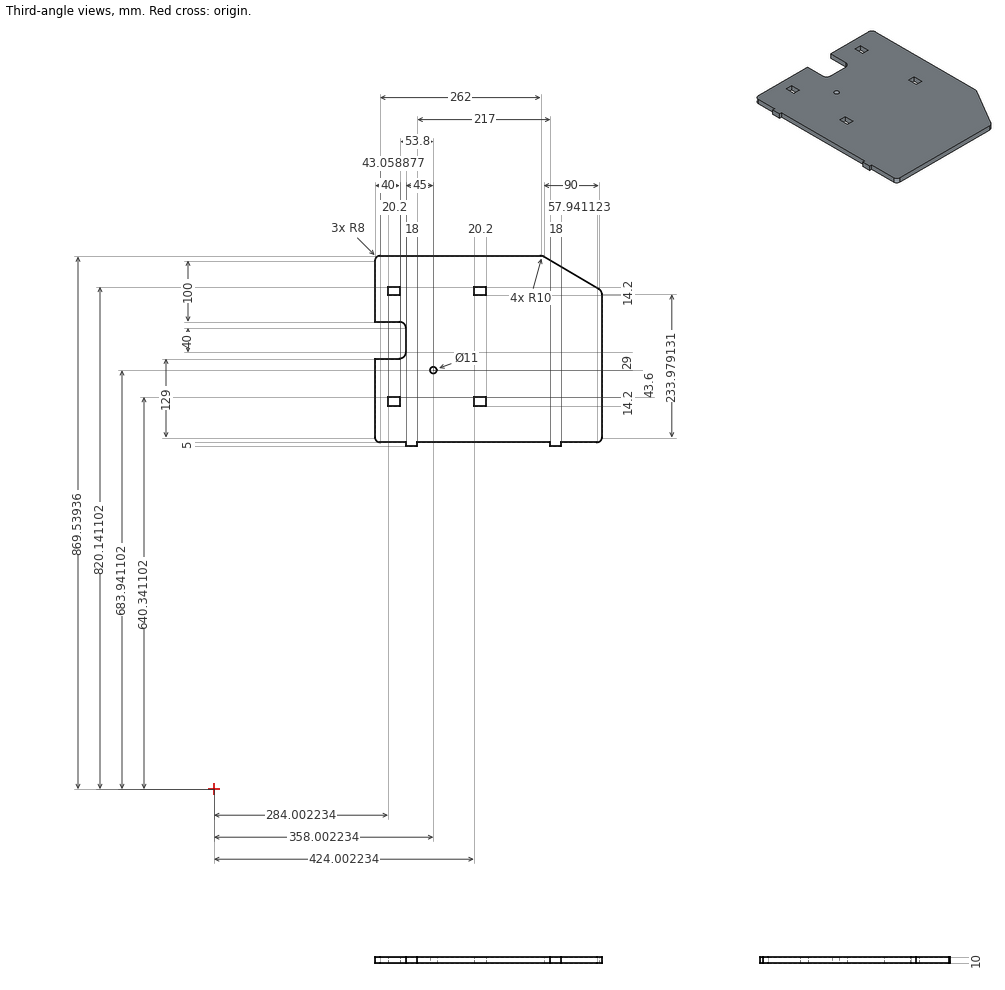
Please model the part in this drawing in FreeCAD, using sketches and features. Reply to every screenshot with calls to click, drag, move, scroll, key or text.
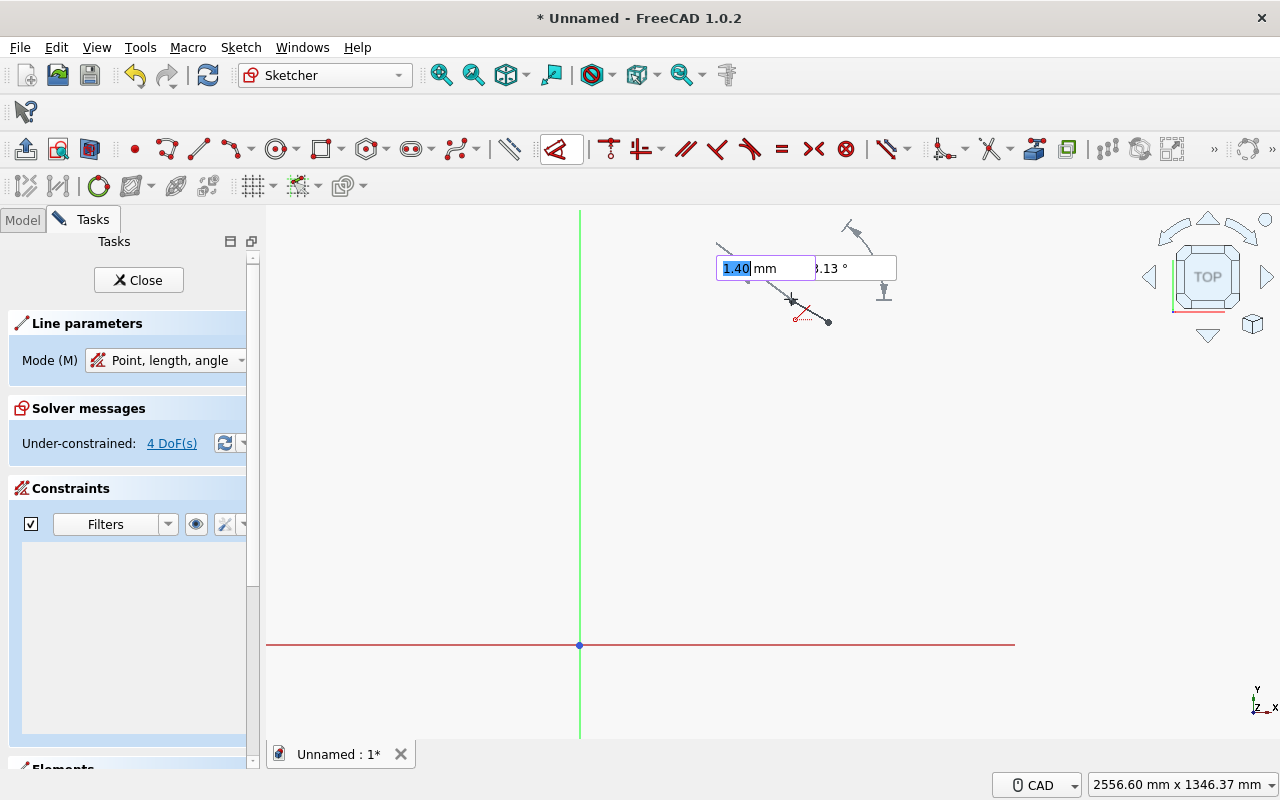
click(687, 300)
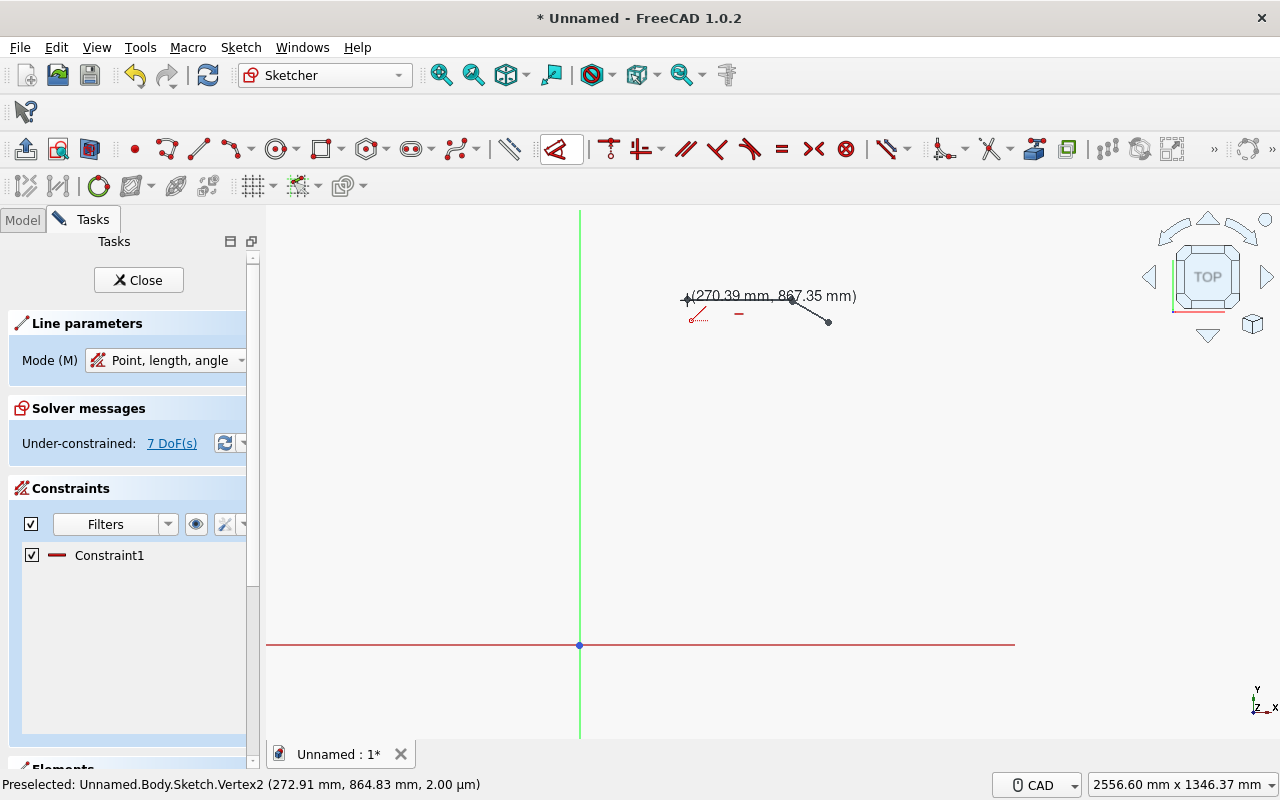
click(168, 150)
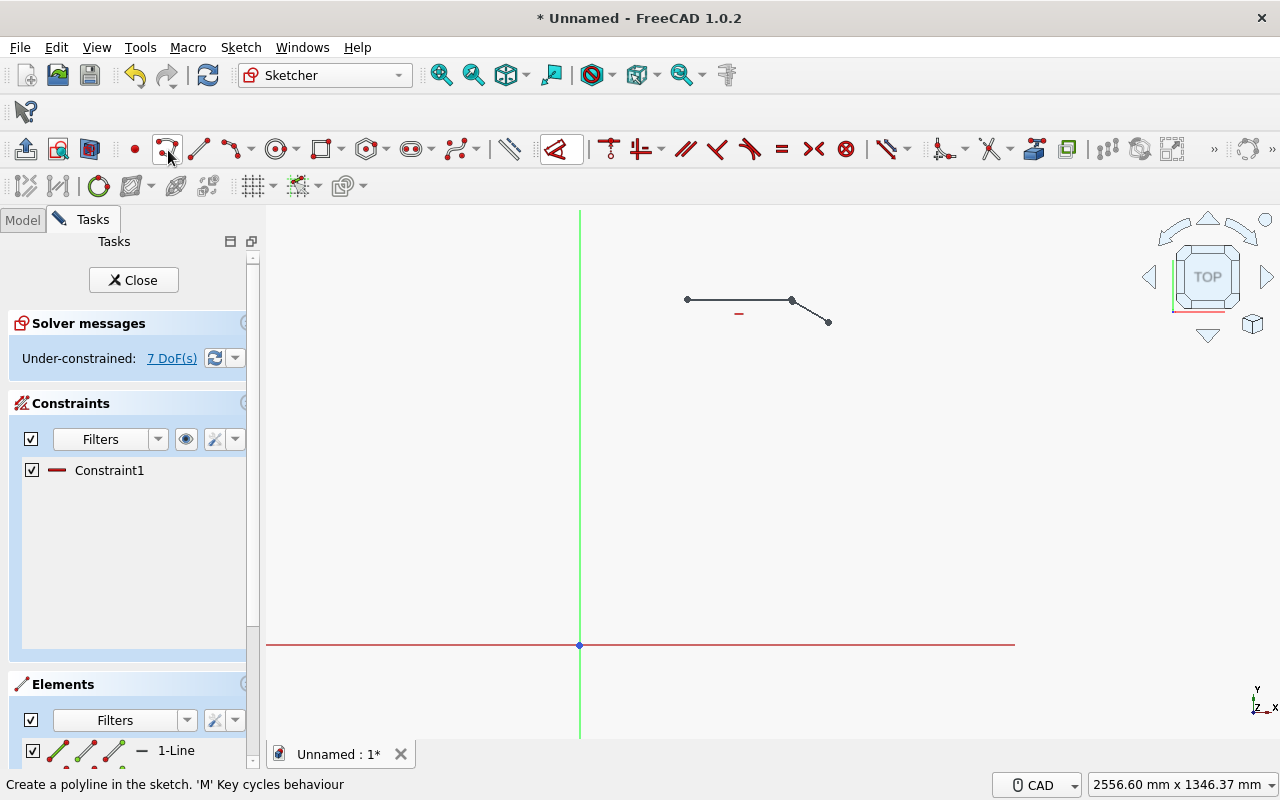
scroll(684, 303, up, 7)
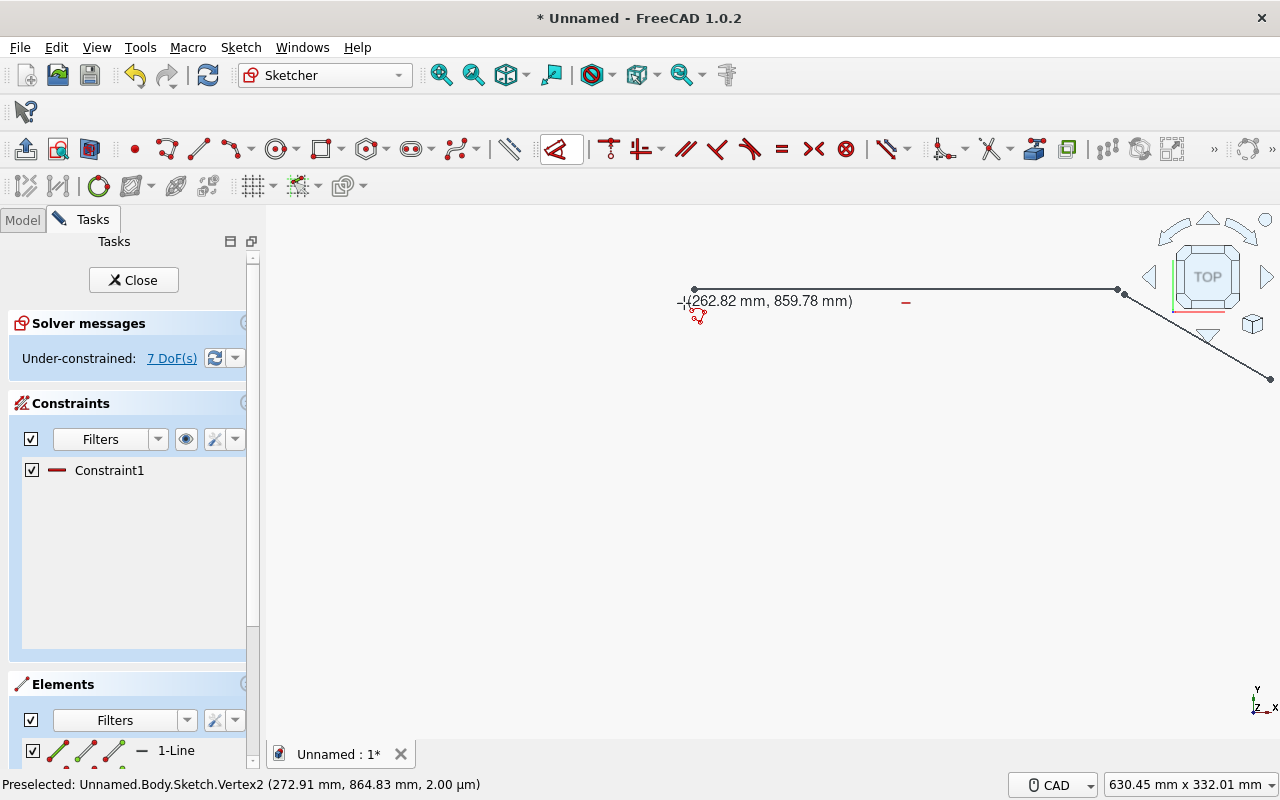
click(683, 301)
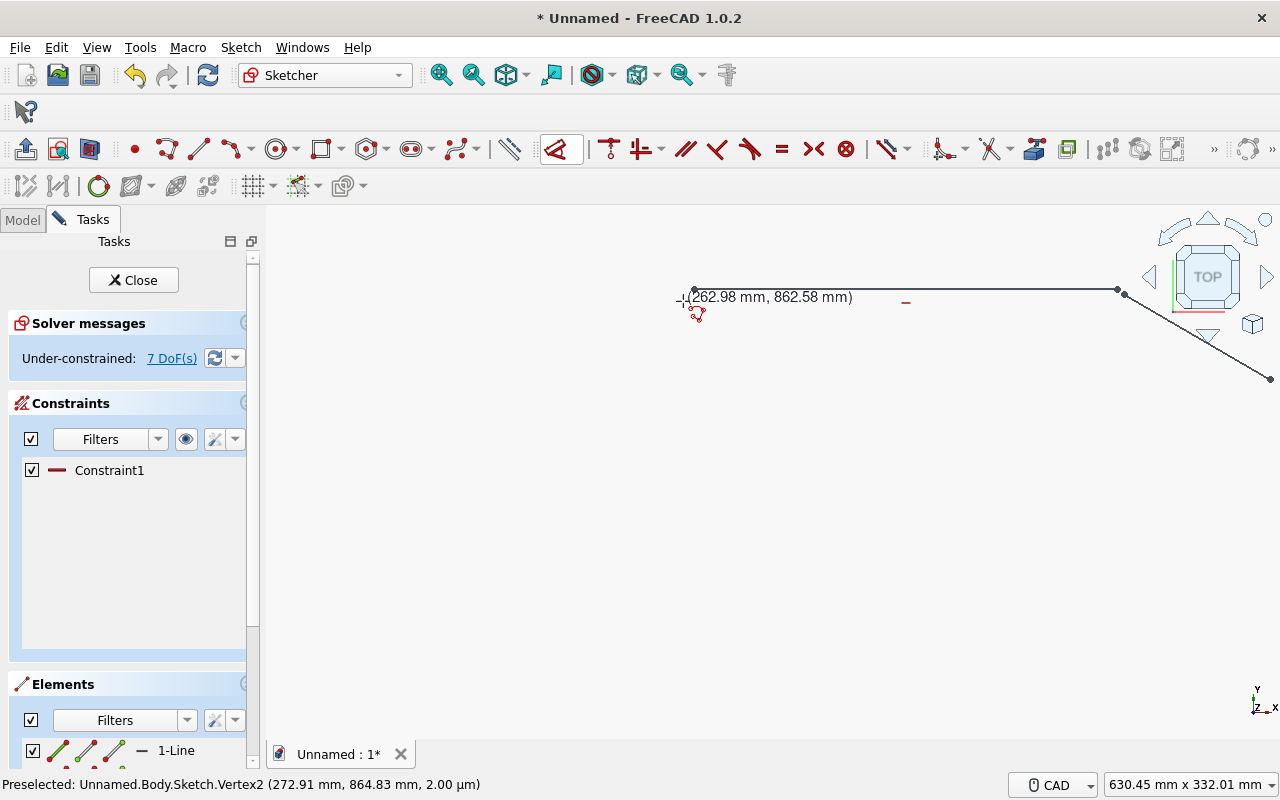
scroll(683, 303, down, 7)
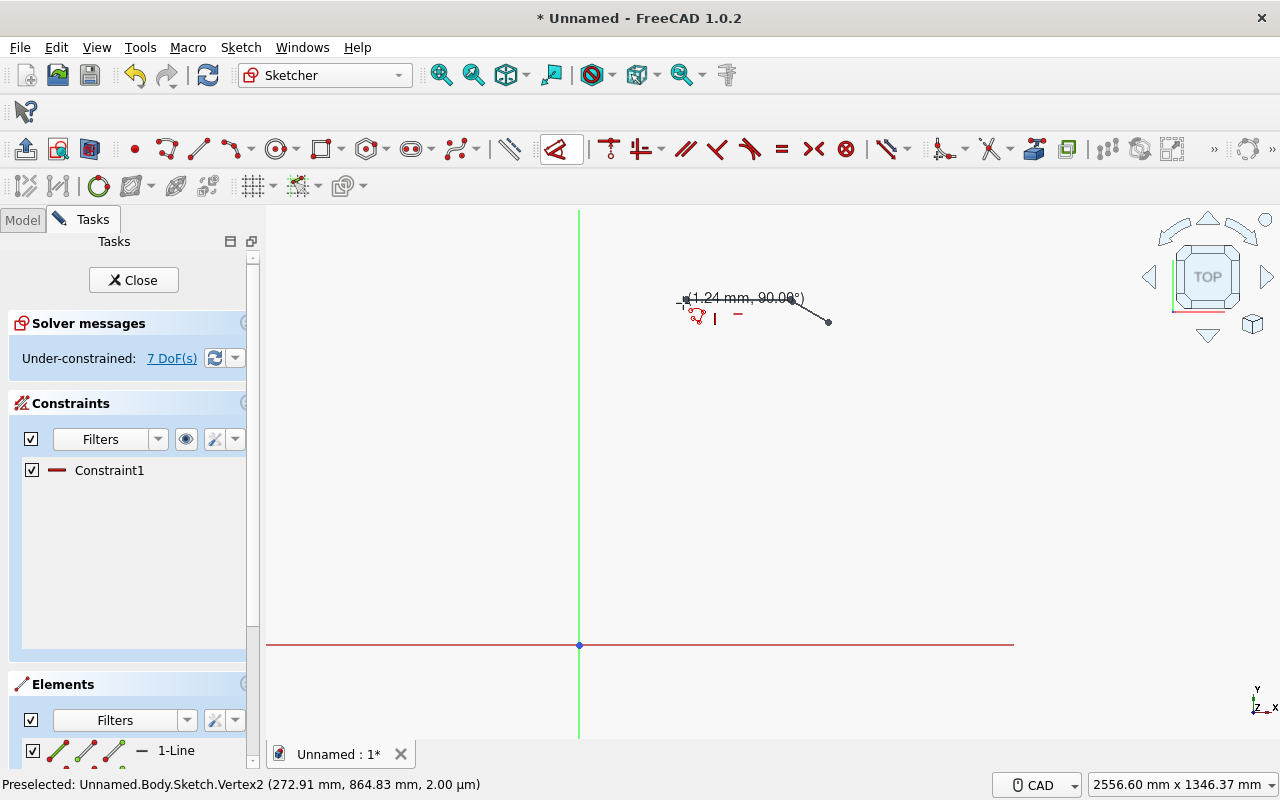
click(683, 342)
click(699, 342)
right_click(699, 342)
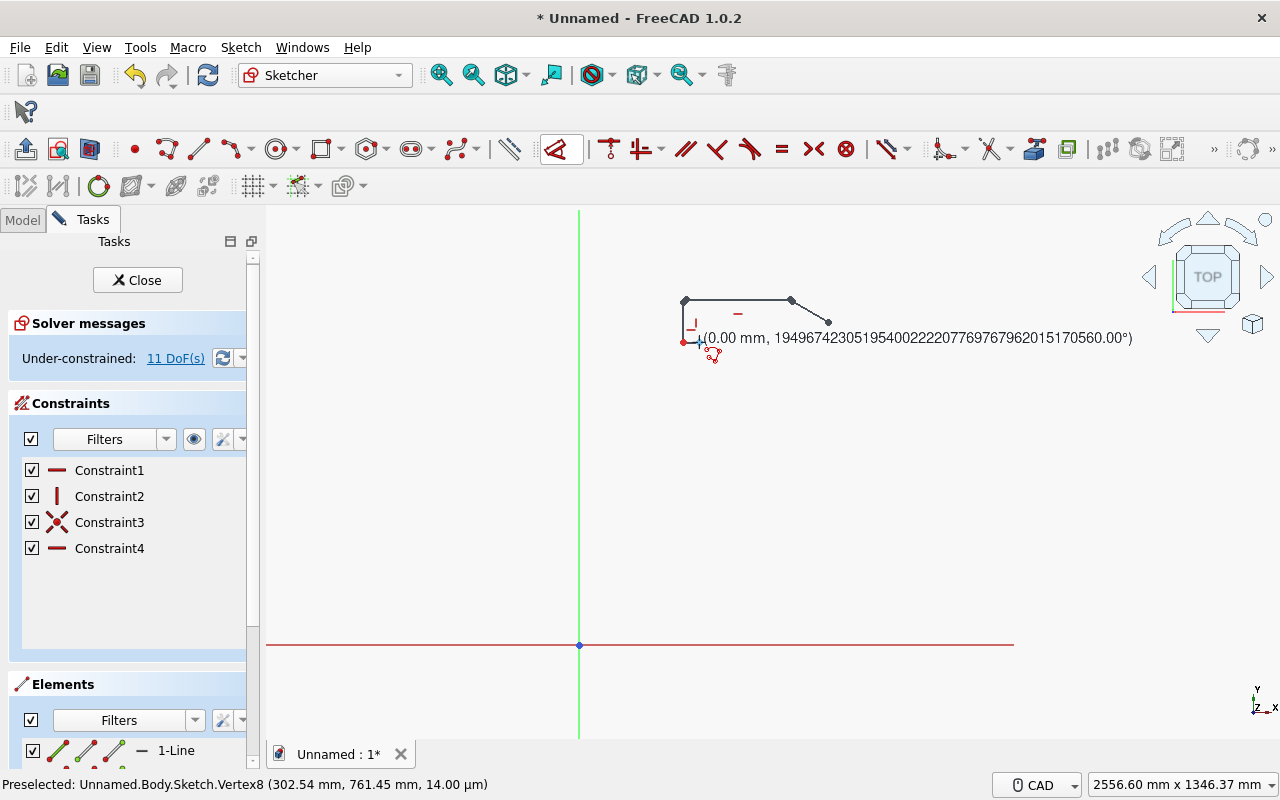
key(g)
key(l)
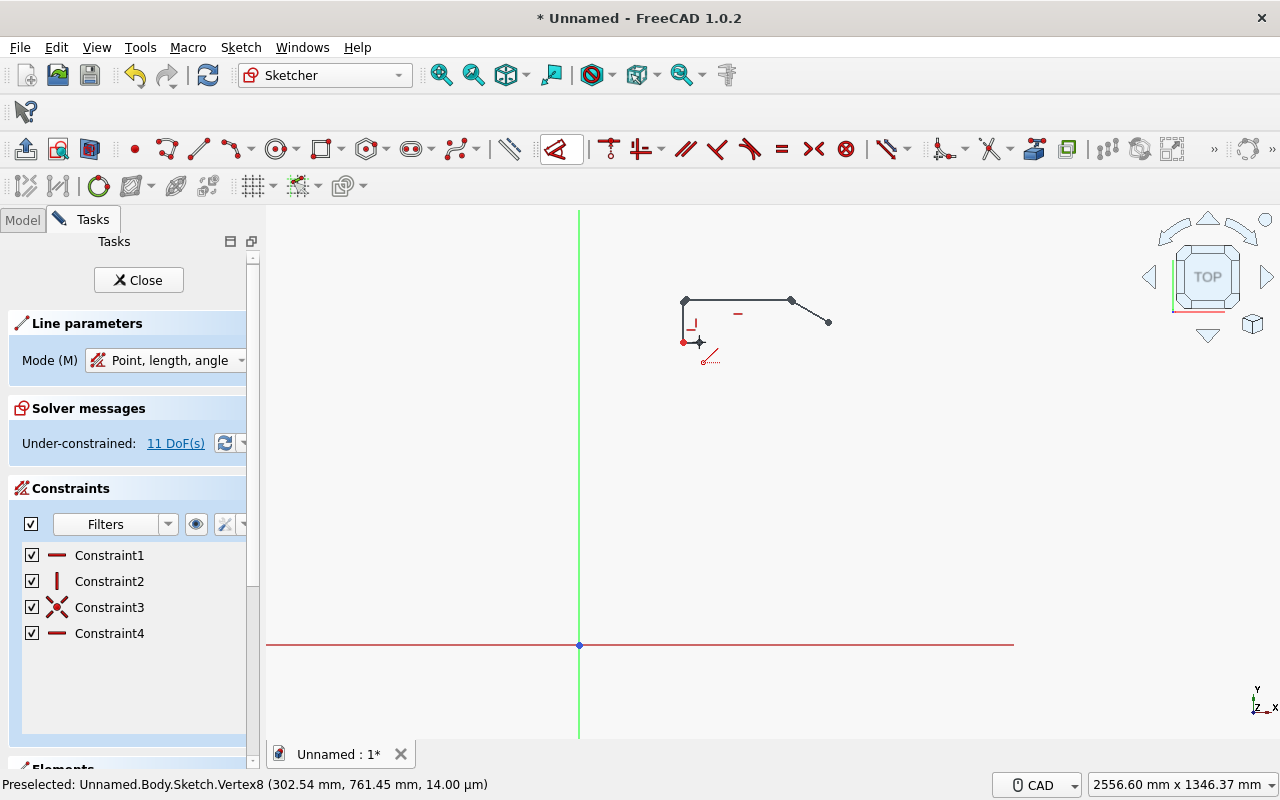
scroll(703, 346, up, 6)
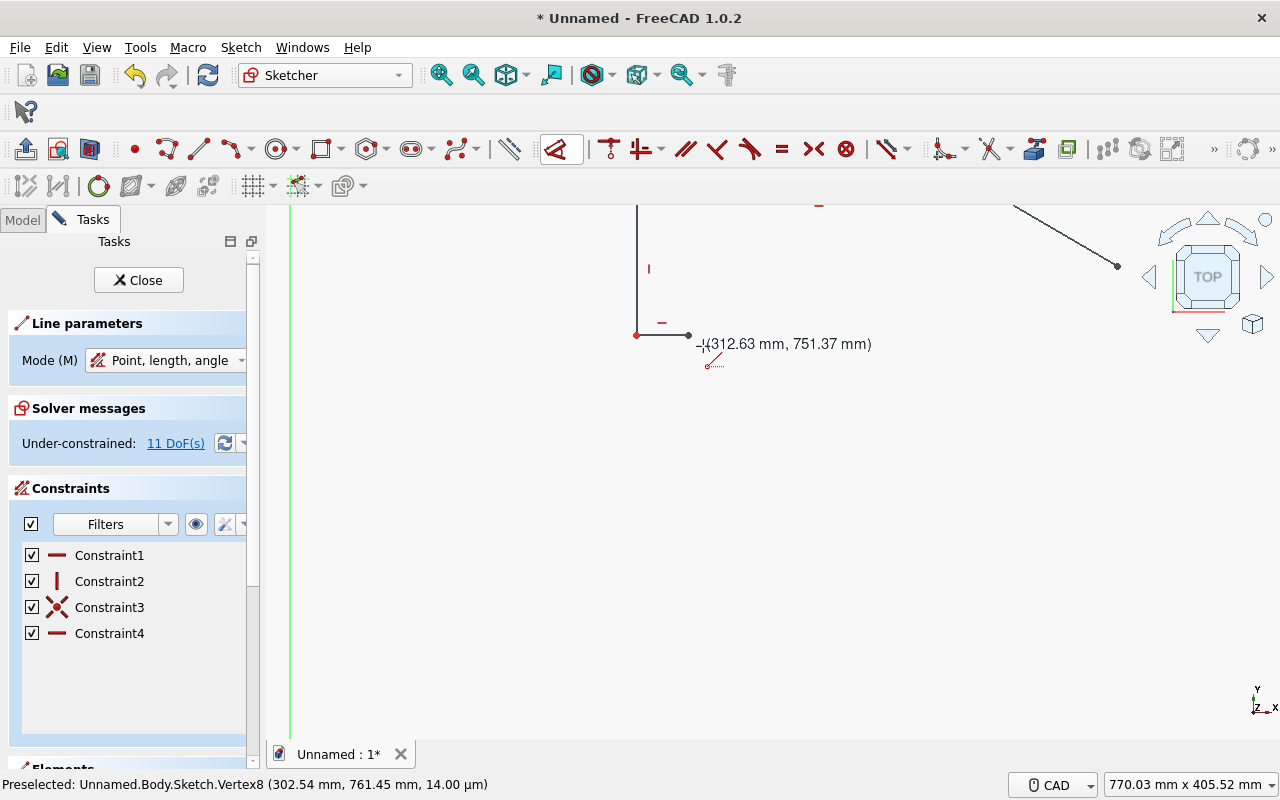
click(702, 347)
click(702, 399)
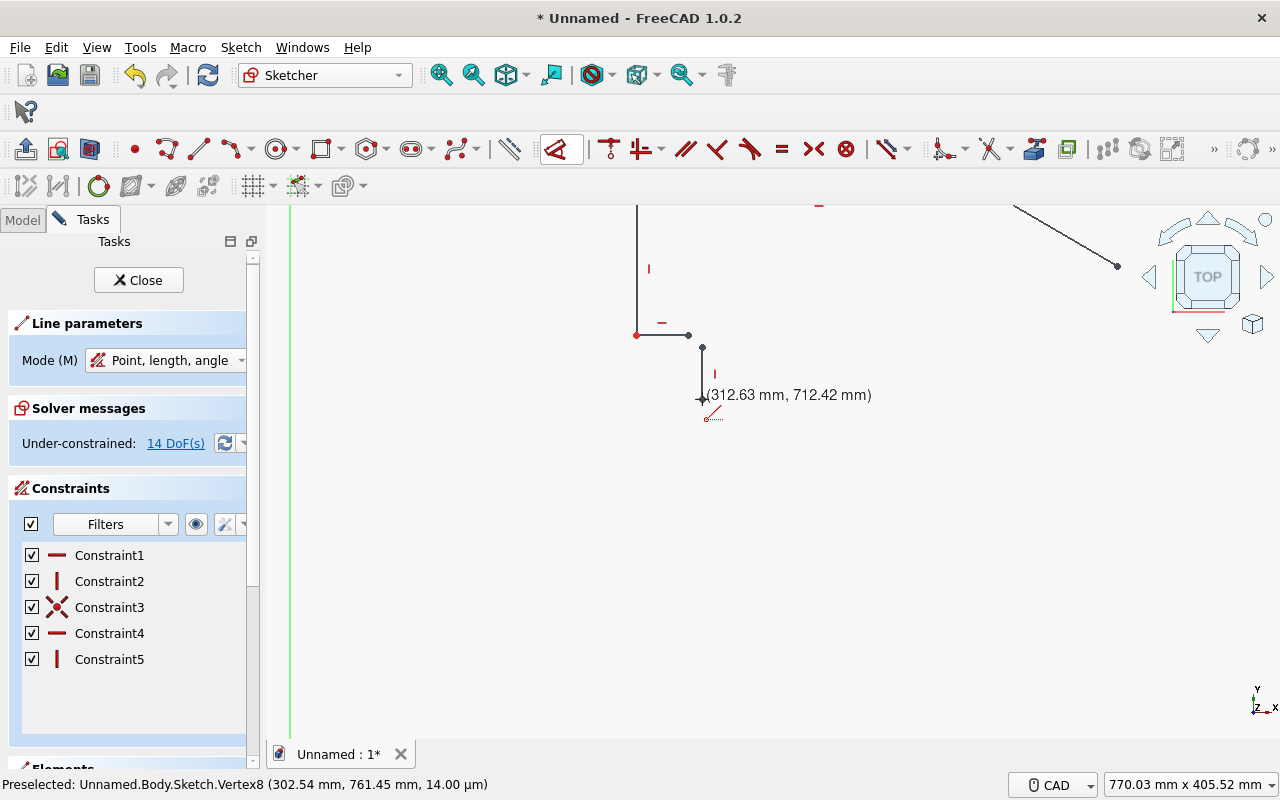
click(168, 150)